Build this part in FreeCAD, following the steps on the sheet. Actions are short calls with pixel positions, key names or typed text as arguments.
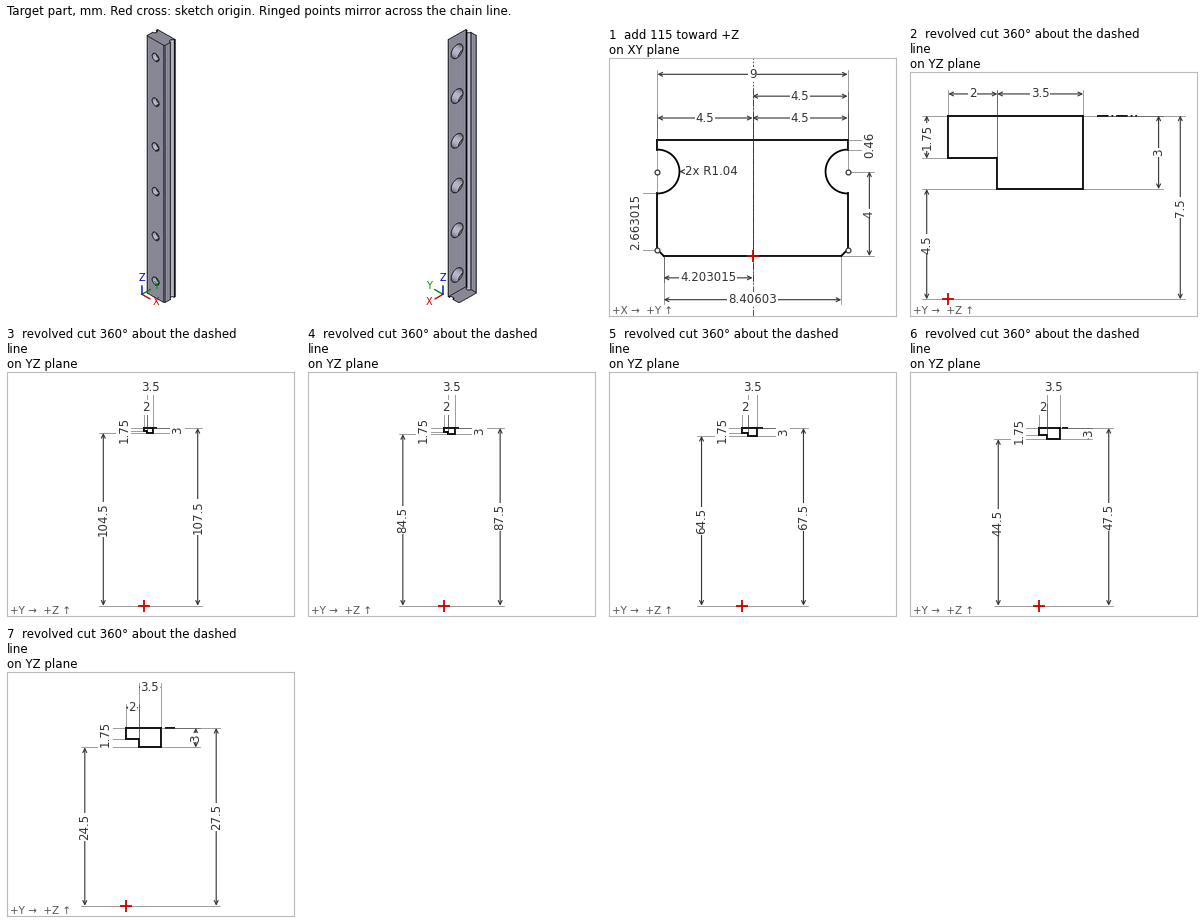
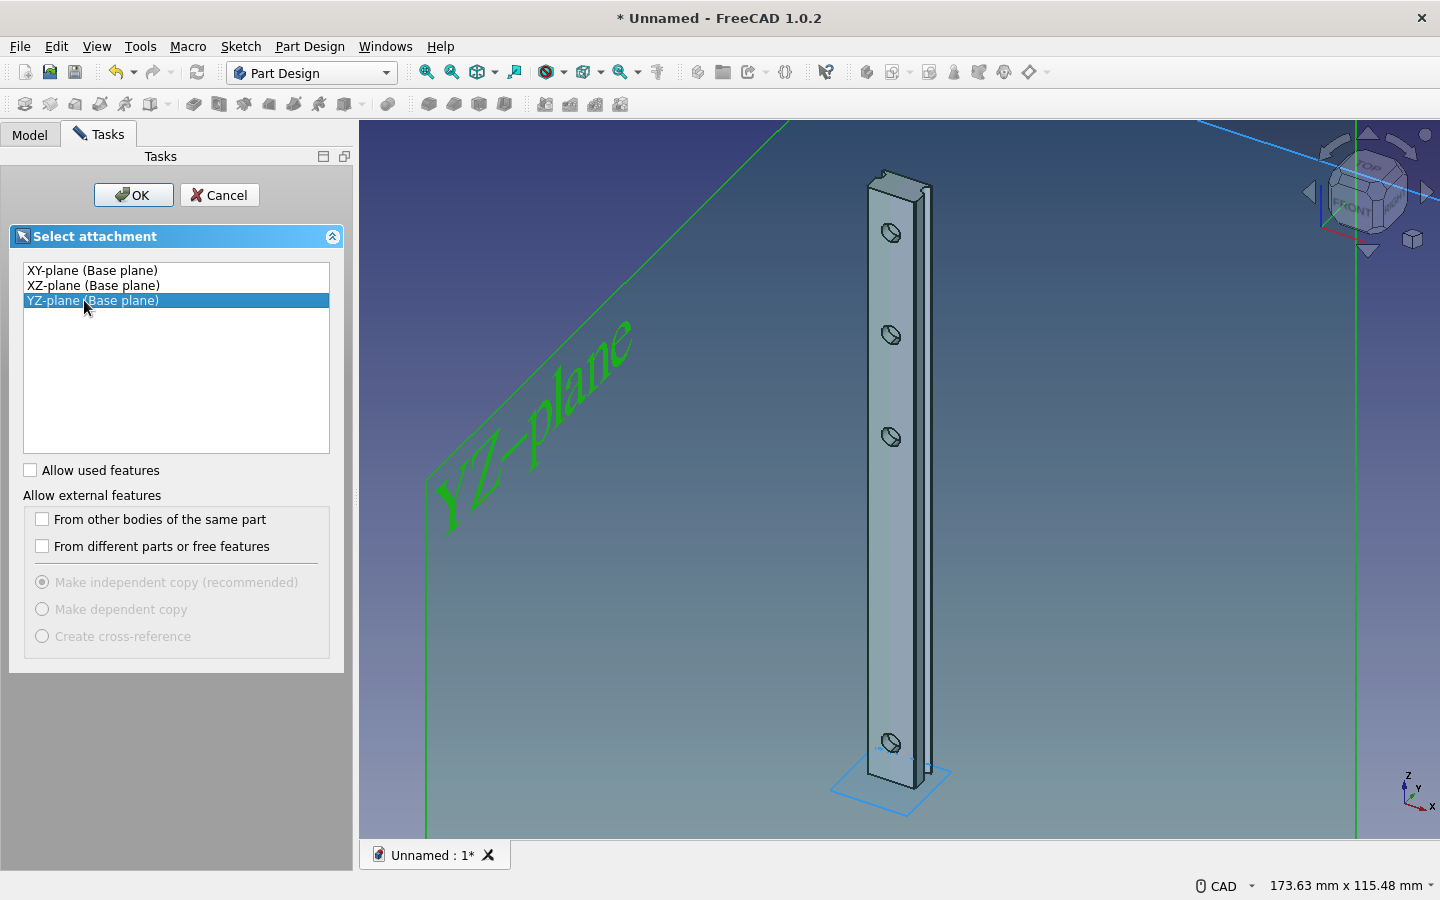
click(134, 195)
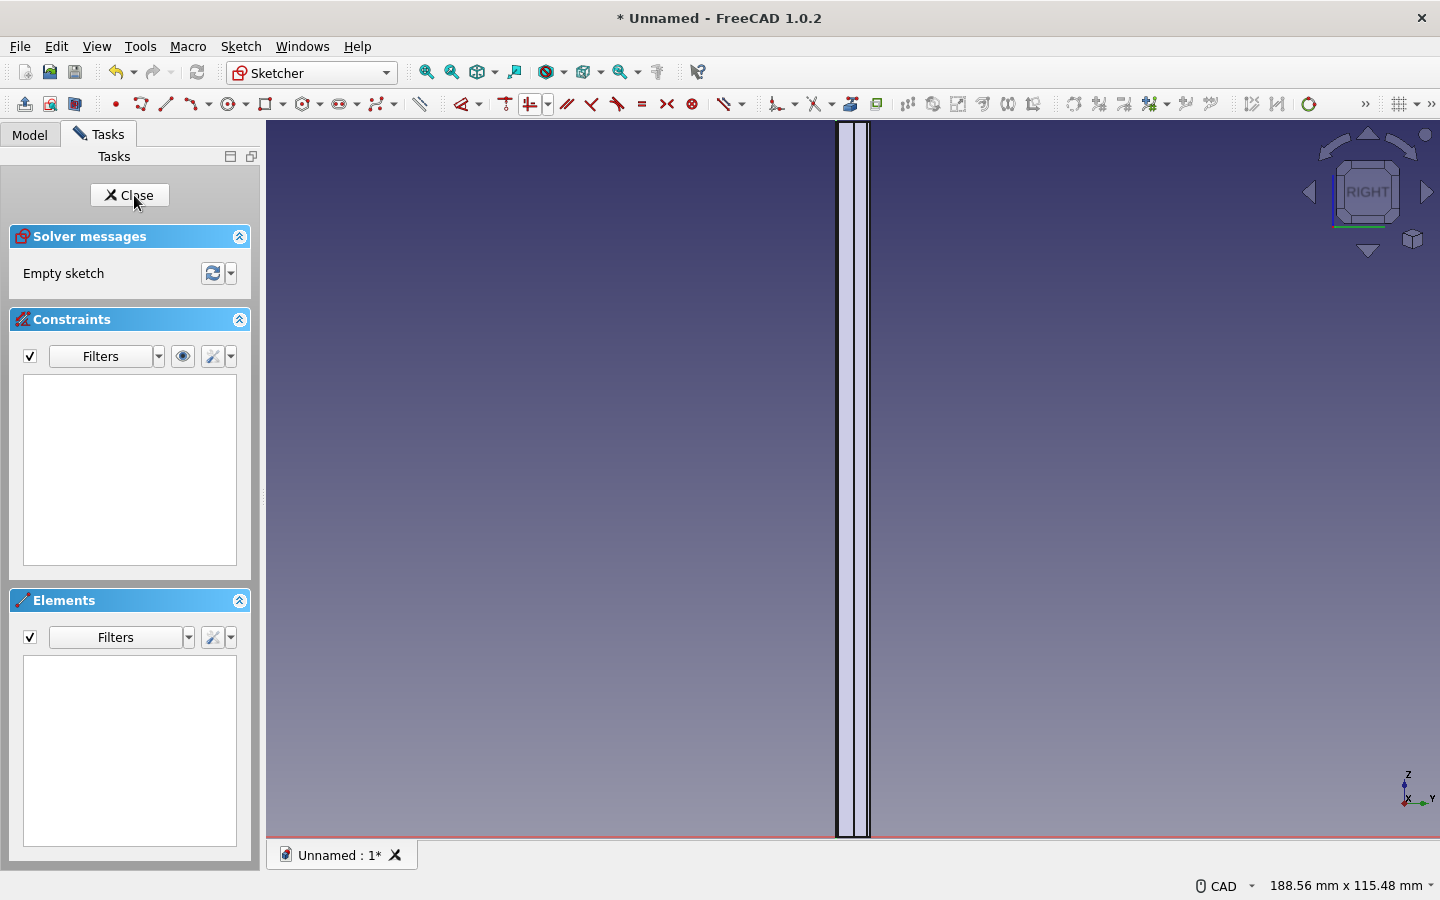
key(q)
key(s)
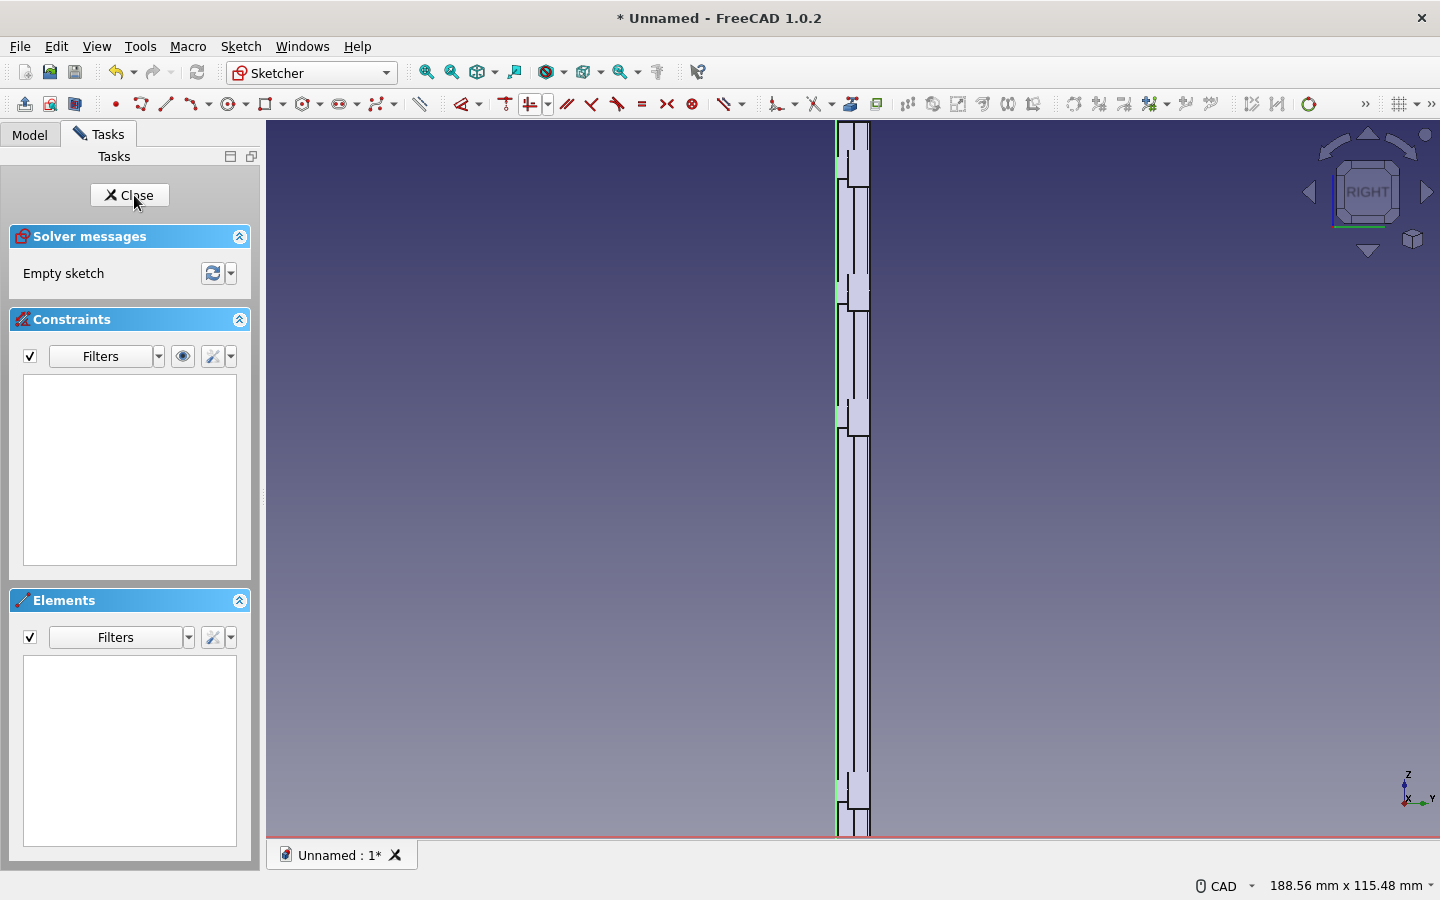
scroll(866, 557, up, 13)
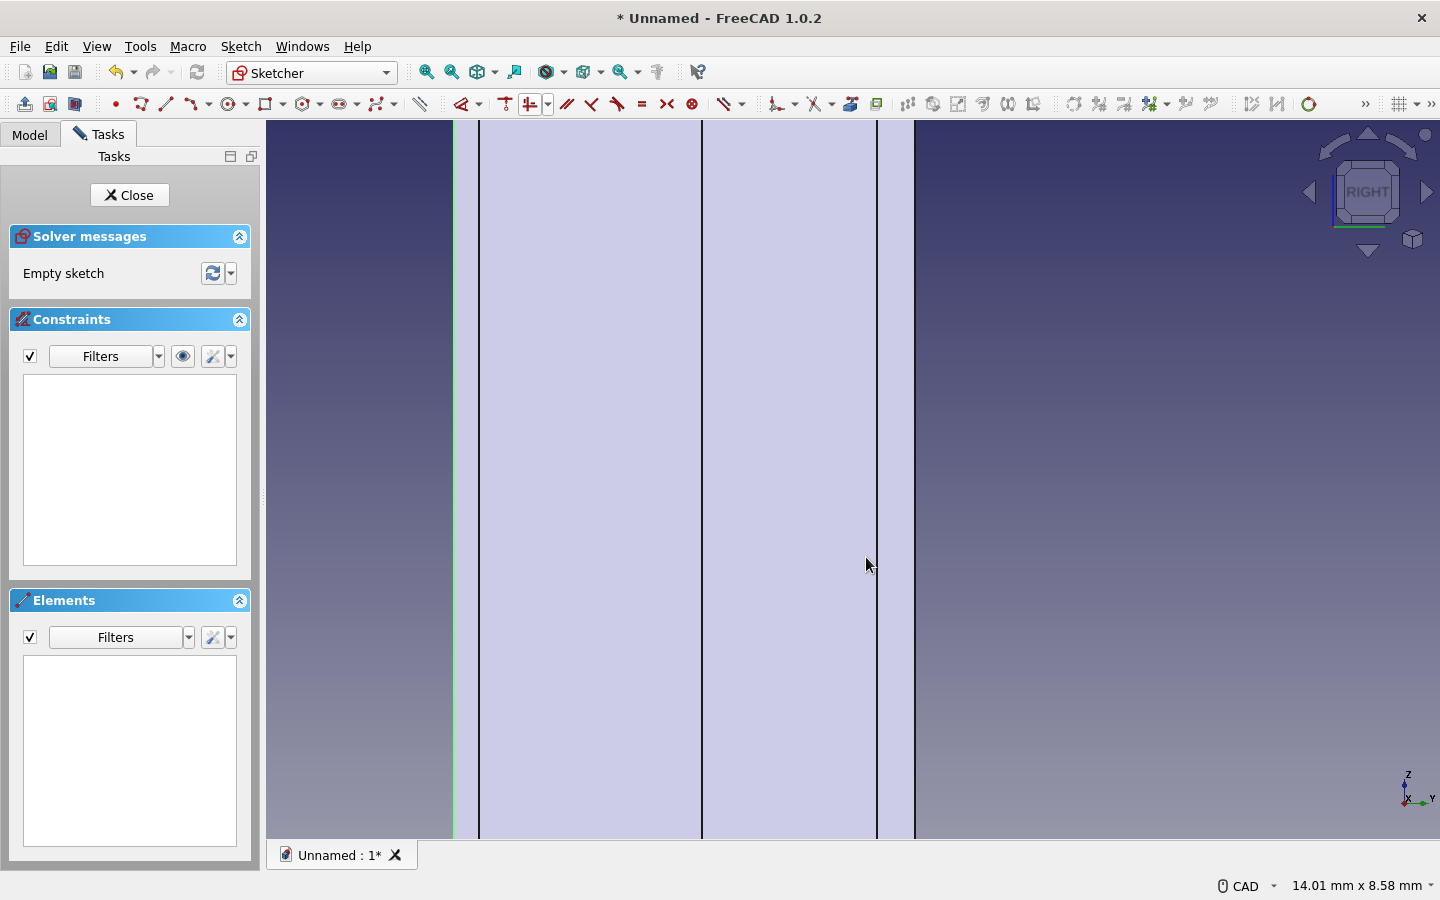
click(141, 104)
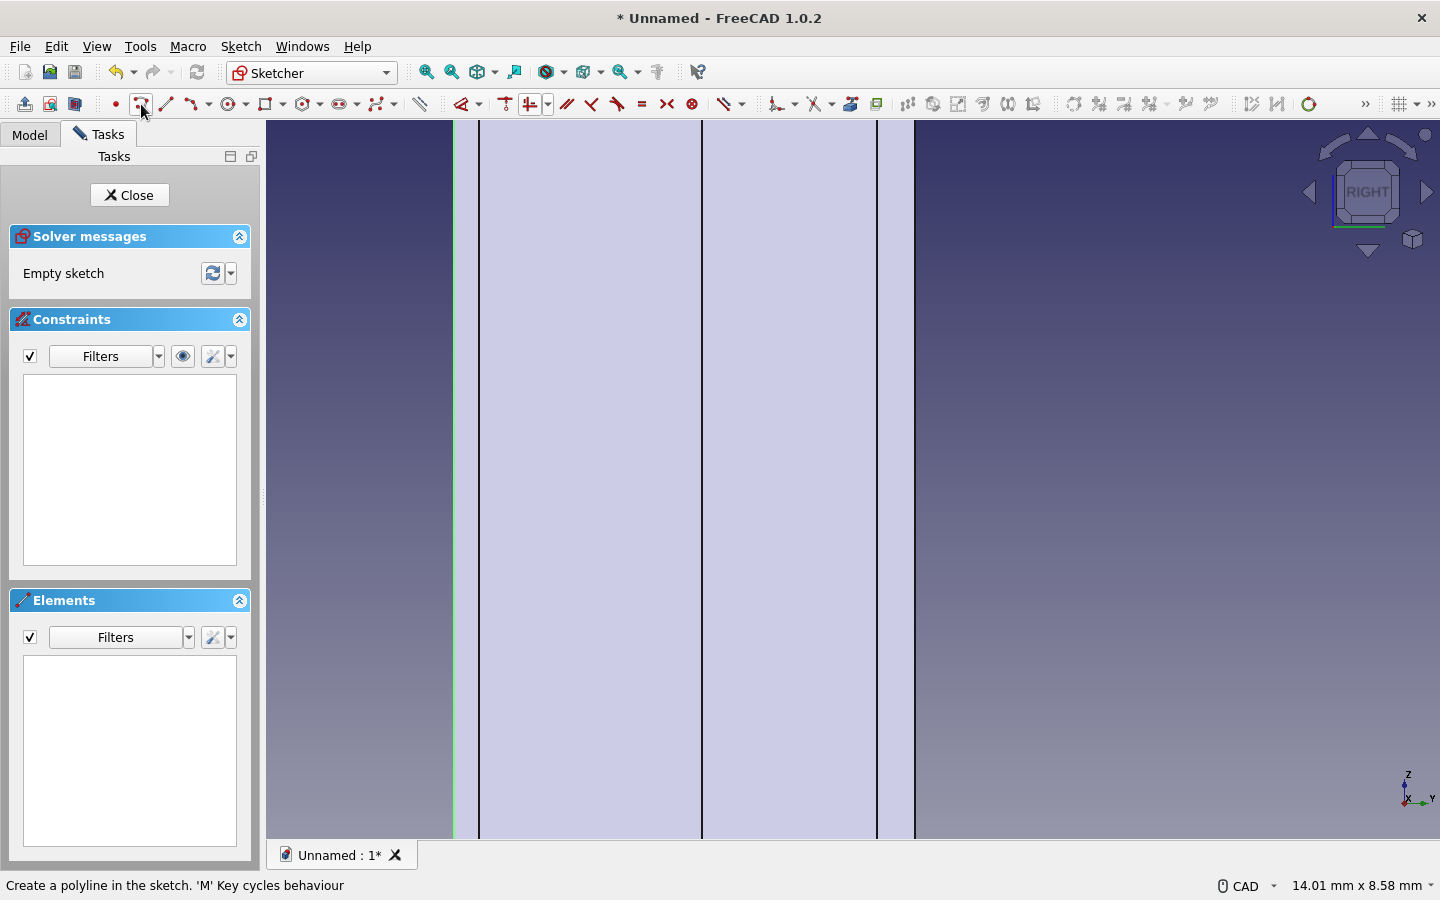
click(622, 596)
click(915, 596)
click(915, 344)
click(454, 344)
click(463, 491)
click(622, 491)
click(622, 597)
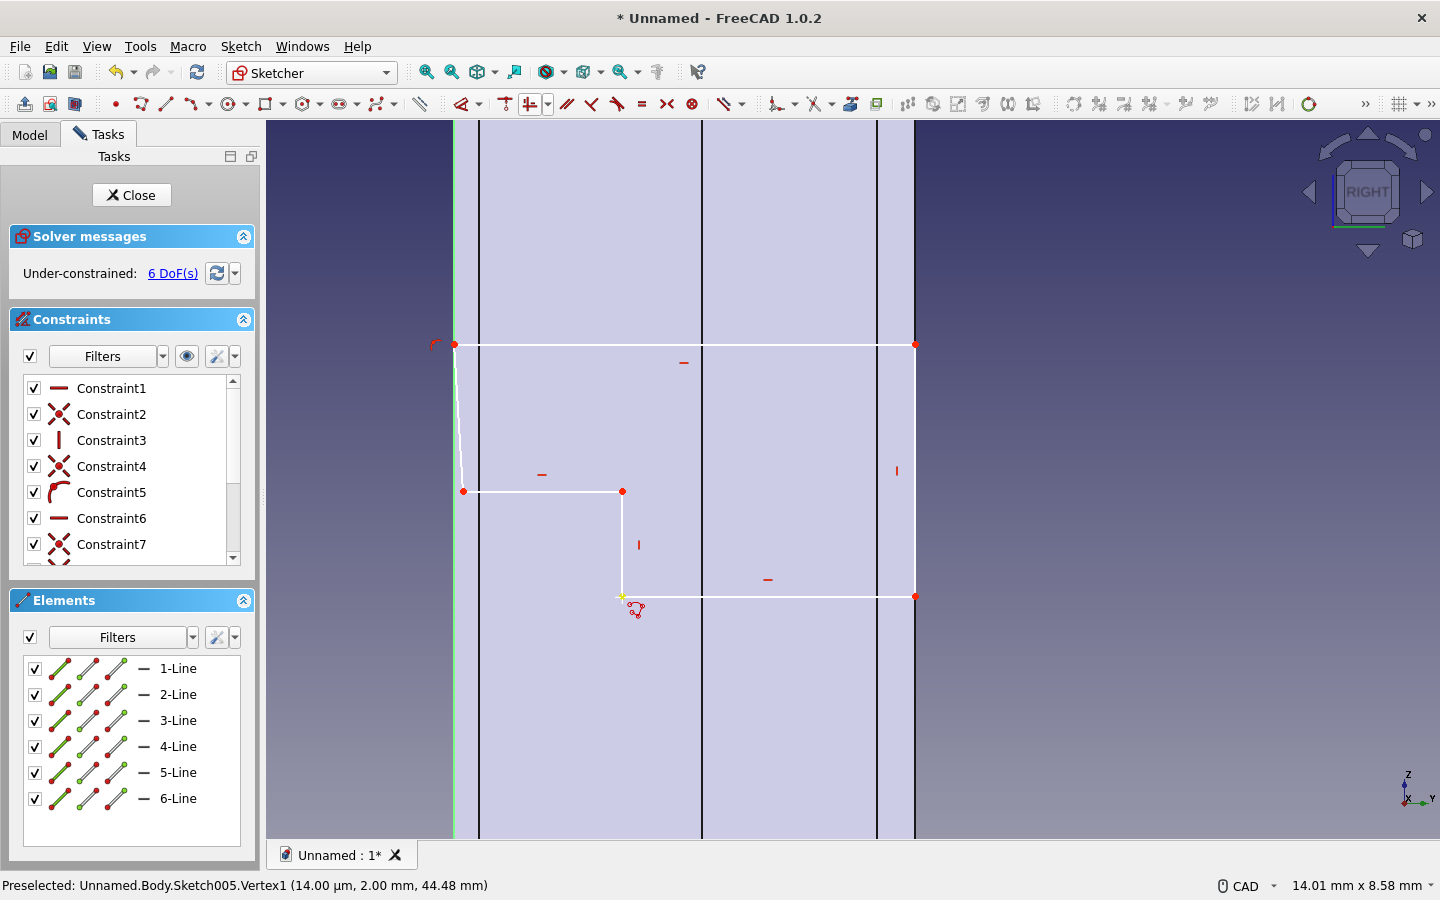
click(166, 104)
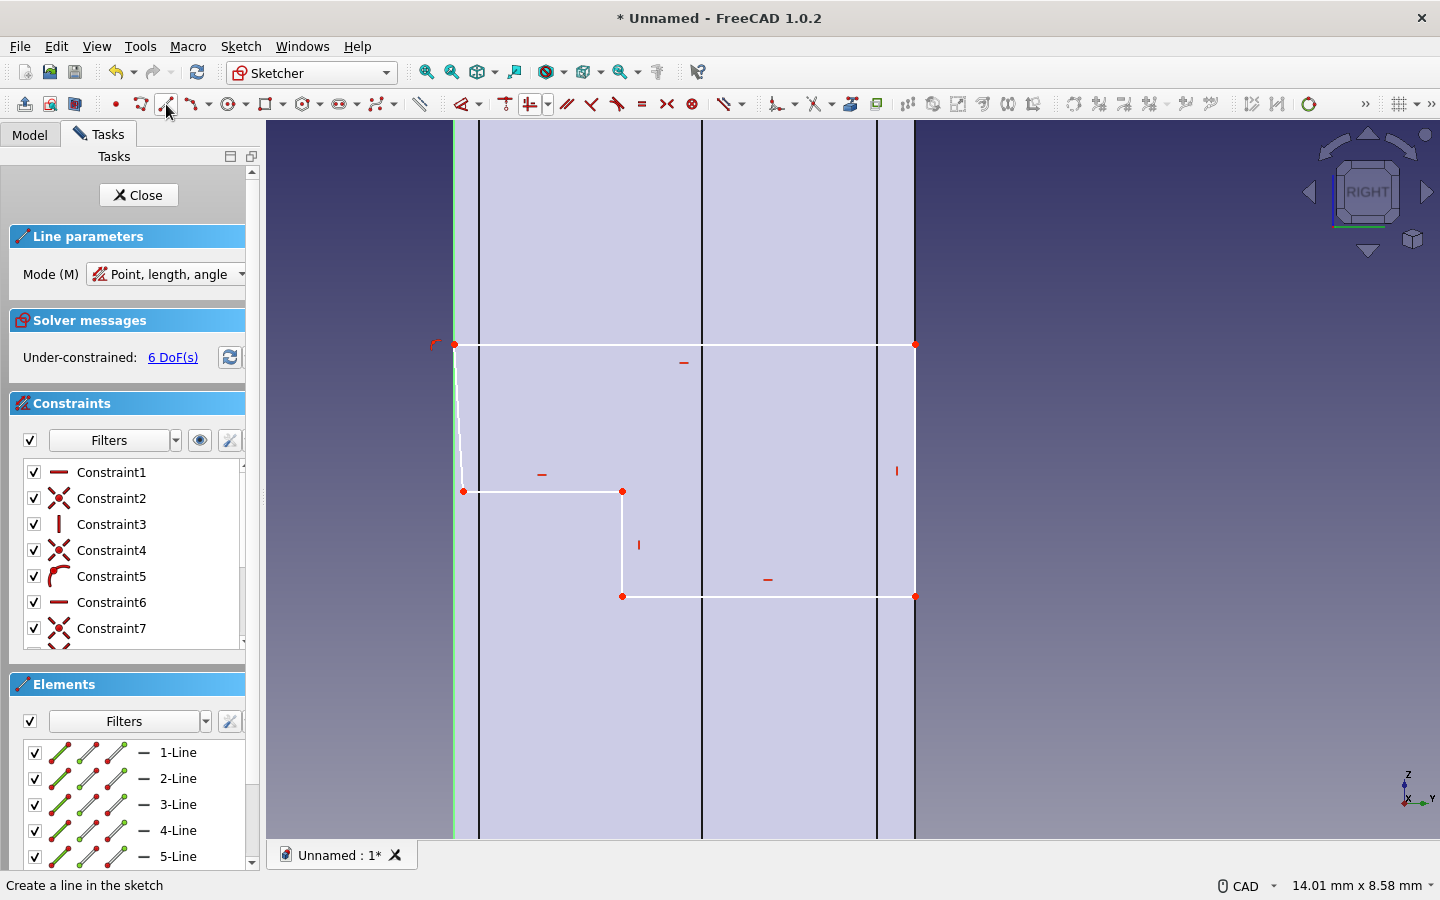
click(961, 344)
click(1100, 344)
key(Escape)